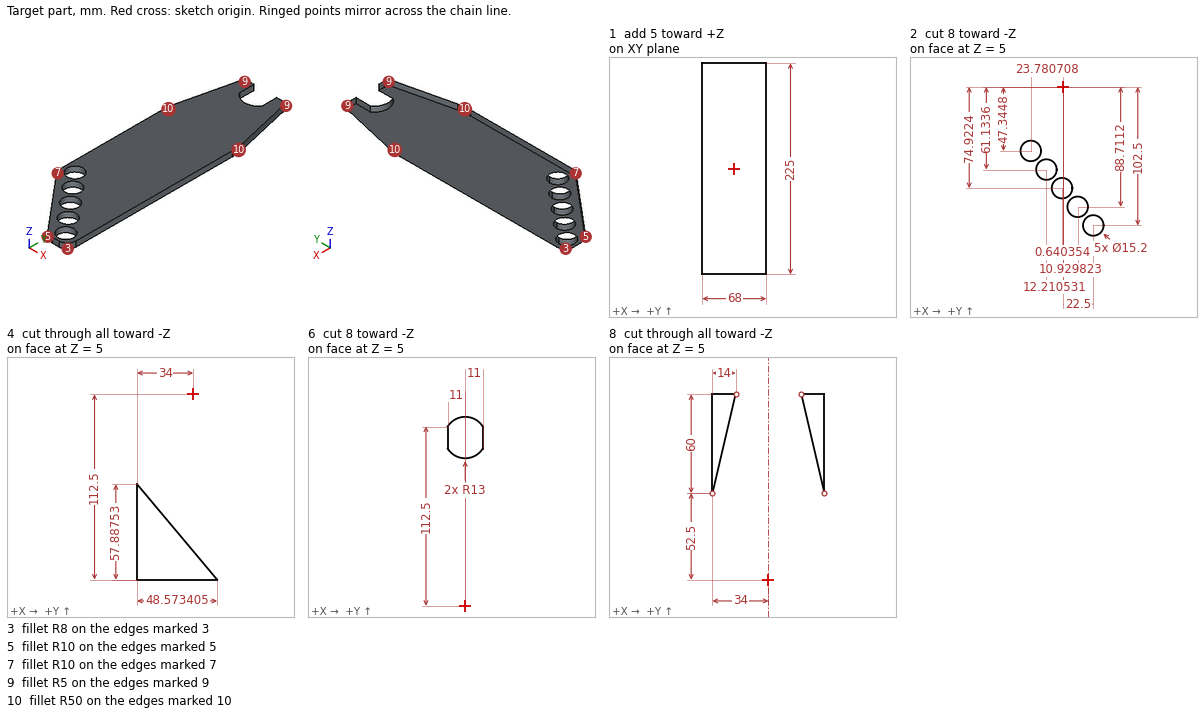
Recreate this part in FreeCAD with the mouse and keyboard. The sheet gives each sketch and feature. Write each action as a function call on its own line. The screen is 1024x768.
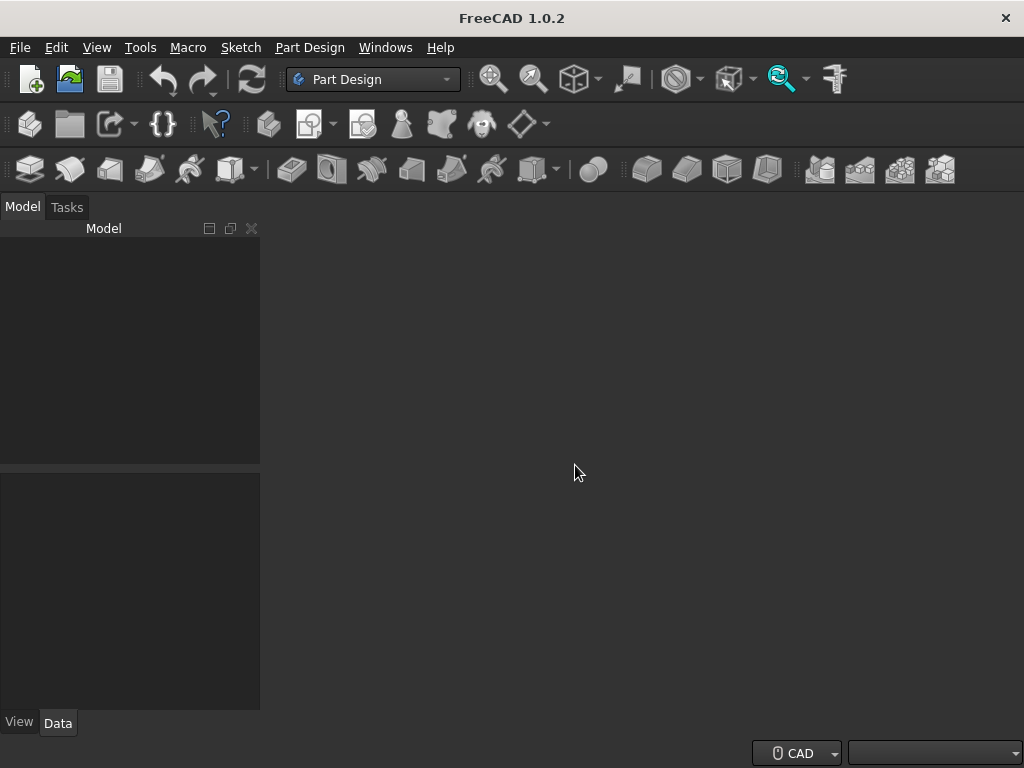
key(ctrl+n)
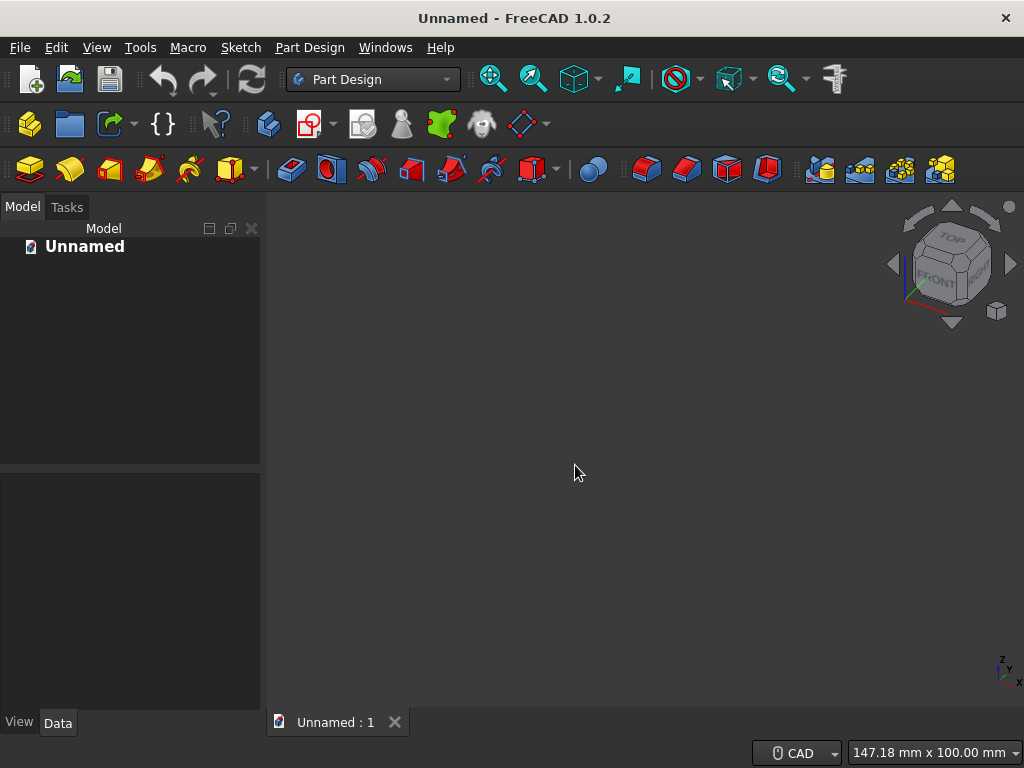
click(310, 124)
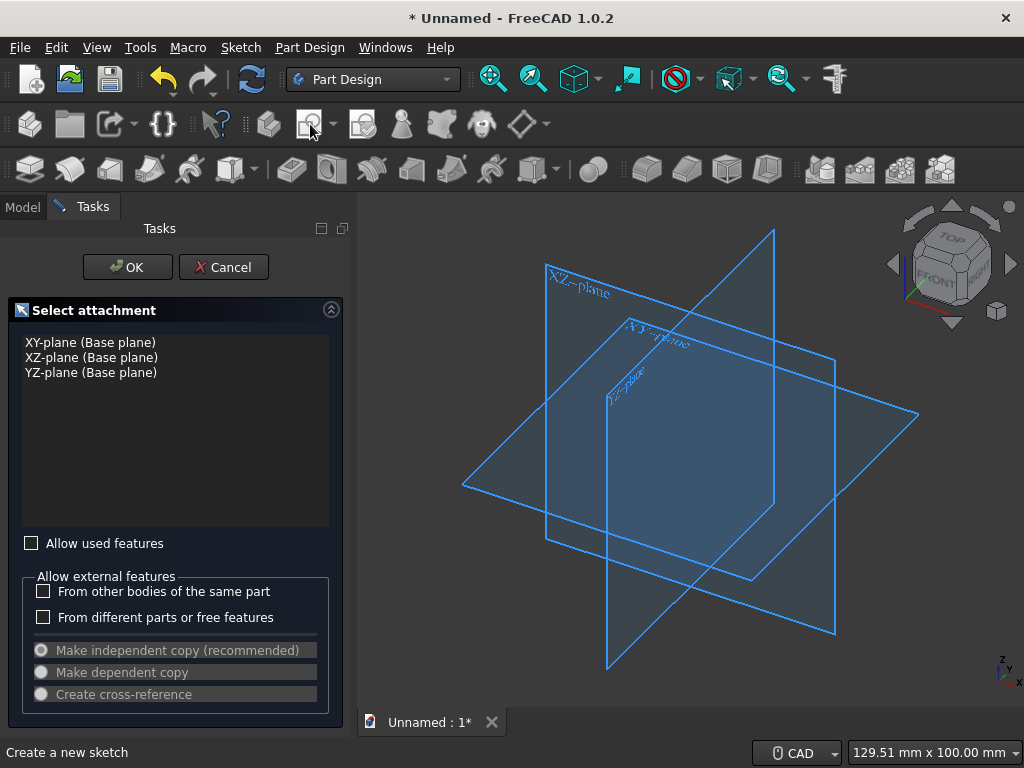
click(82, 342)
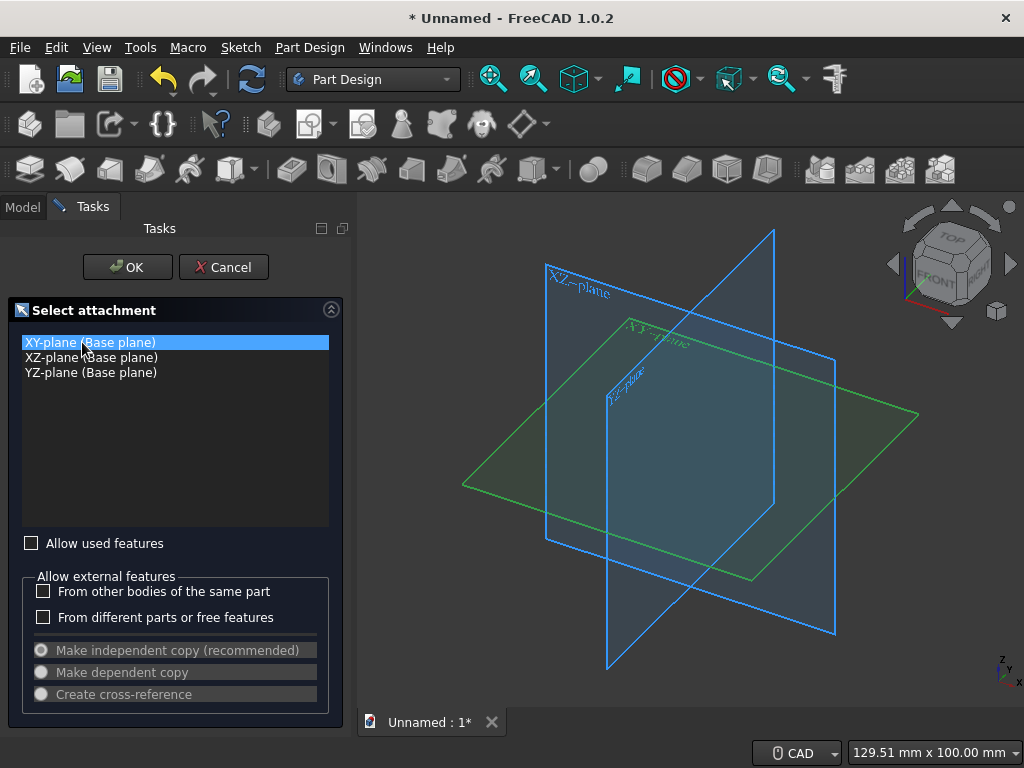
click(128, 267)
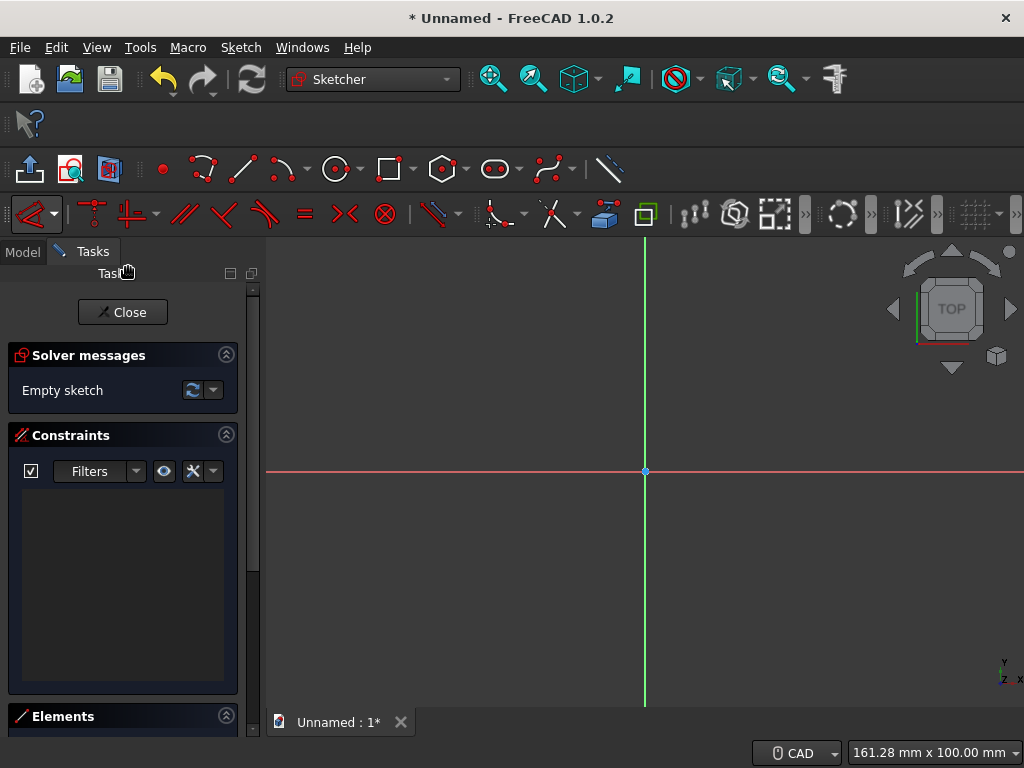
scroll(547, 472, down, 6)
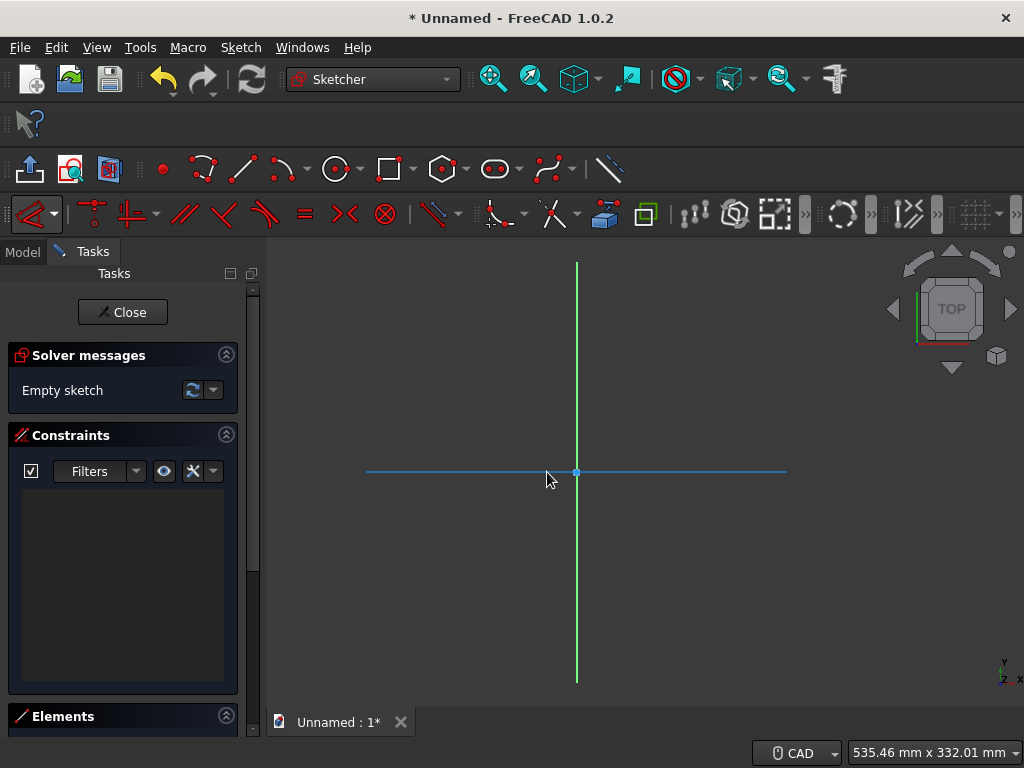
key(g)
key(v)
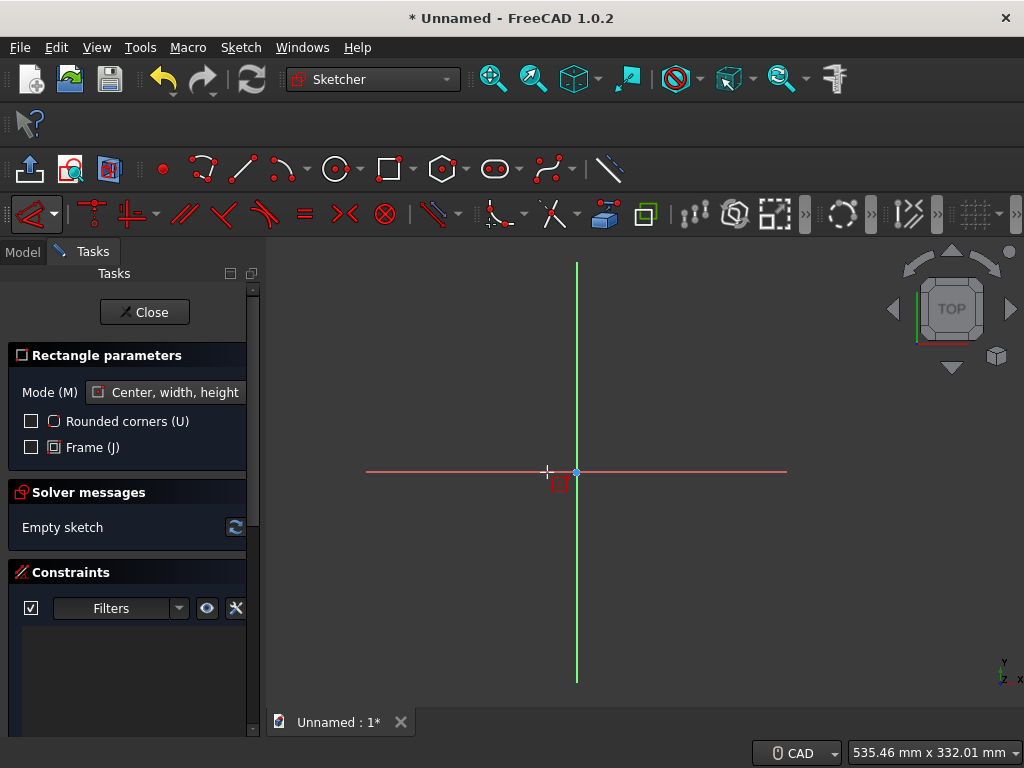
click(577, 472)
click(625, 313)
key(Escape)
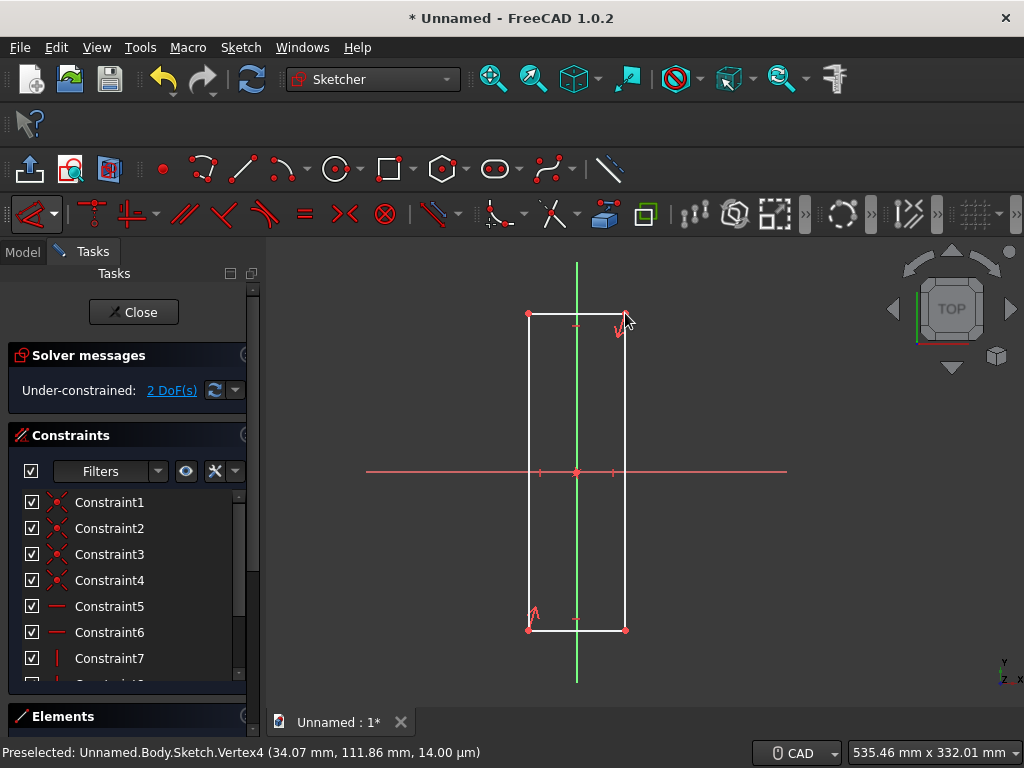
key(d)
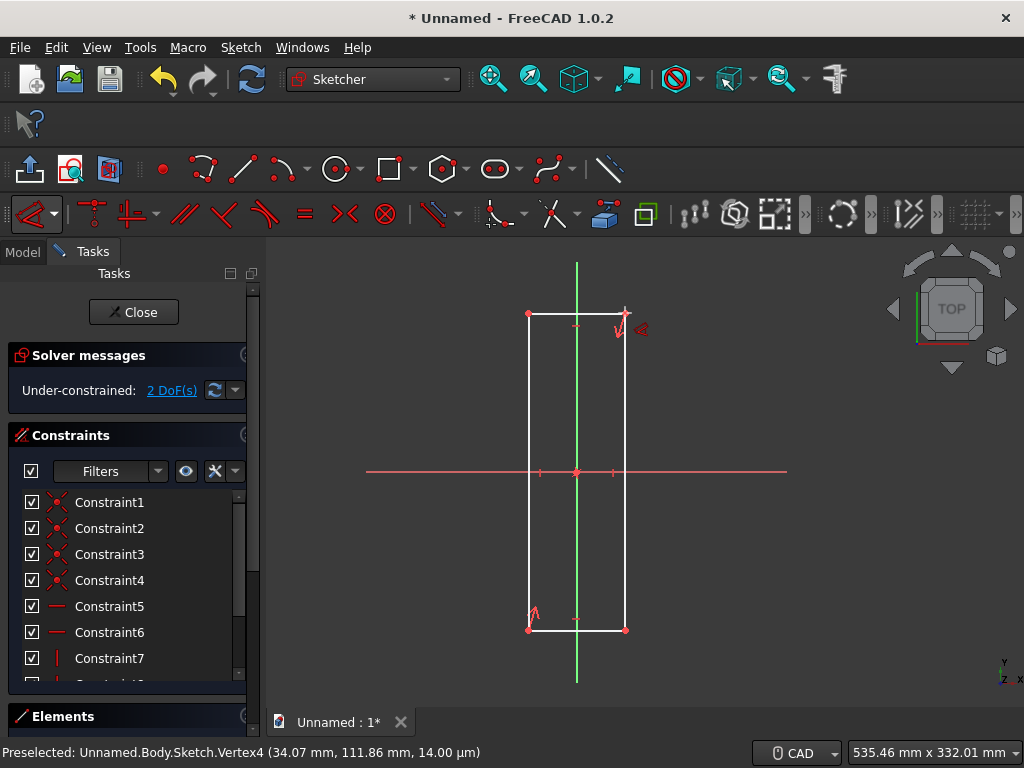
click(557, 631)
click(555, 665)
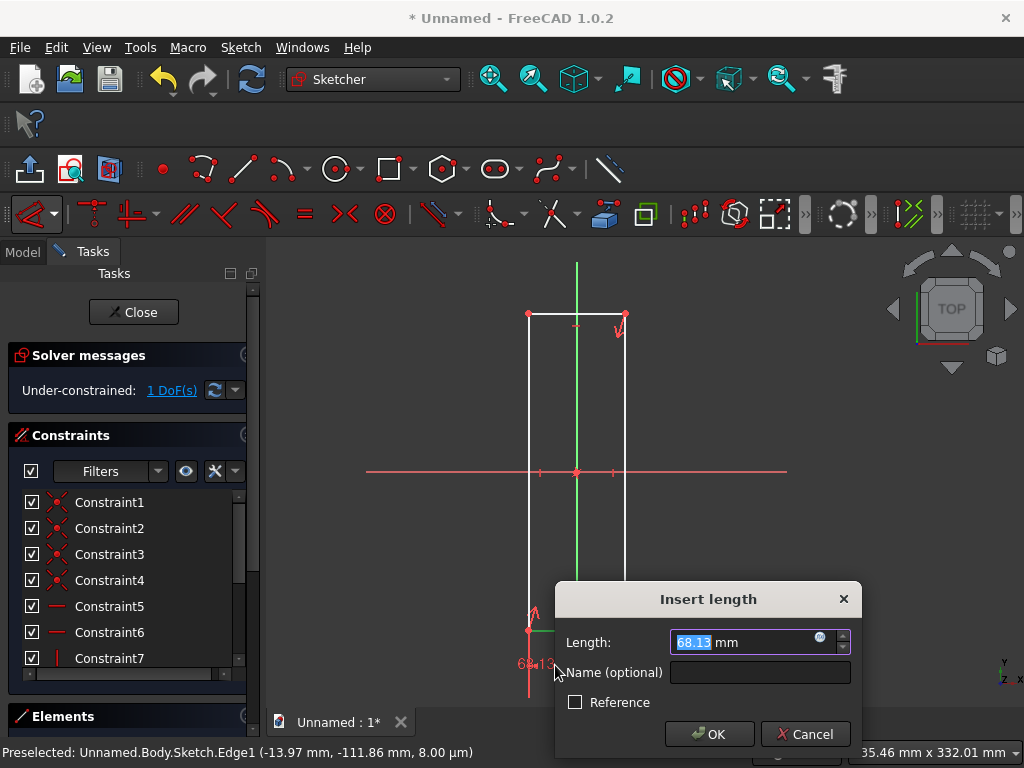
text(68)
key(Return)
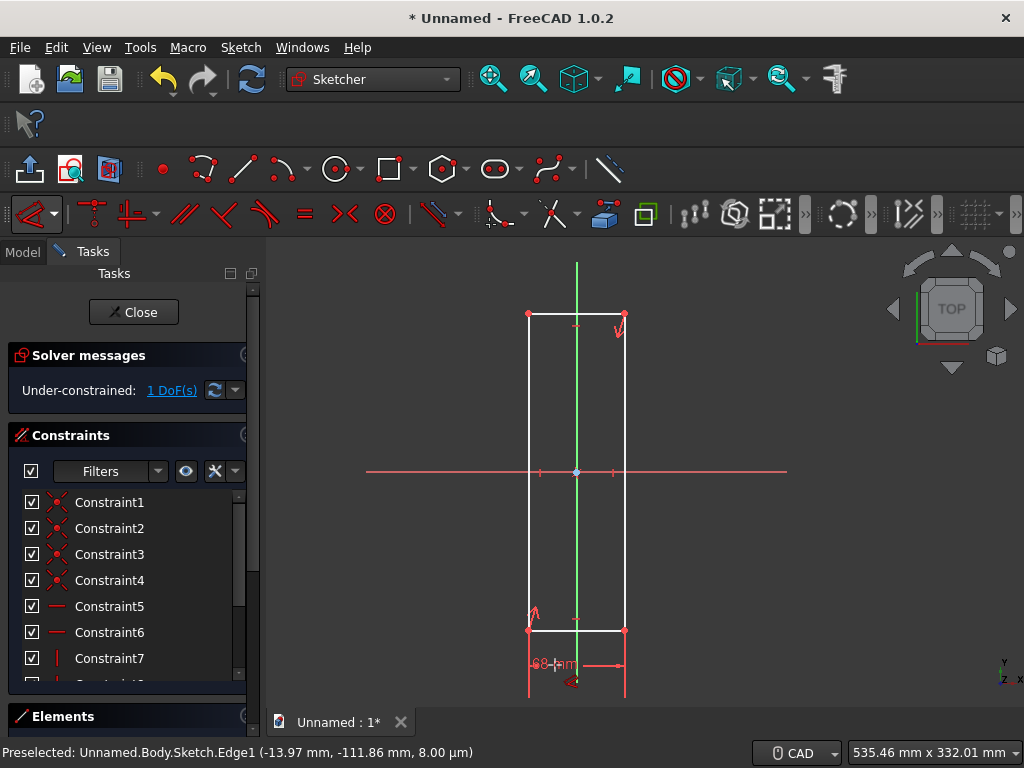
click(625, 536)
click(659, 400)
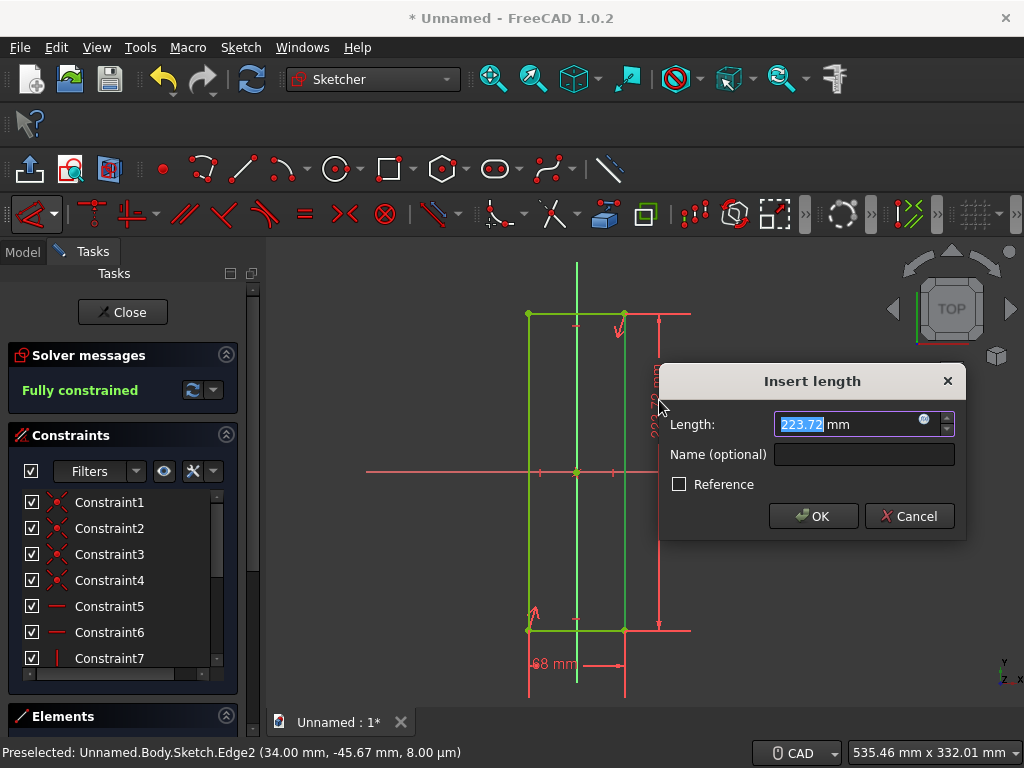
text(225)
key(Return)
key(Escape)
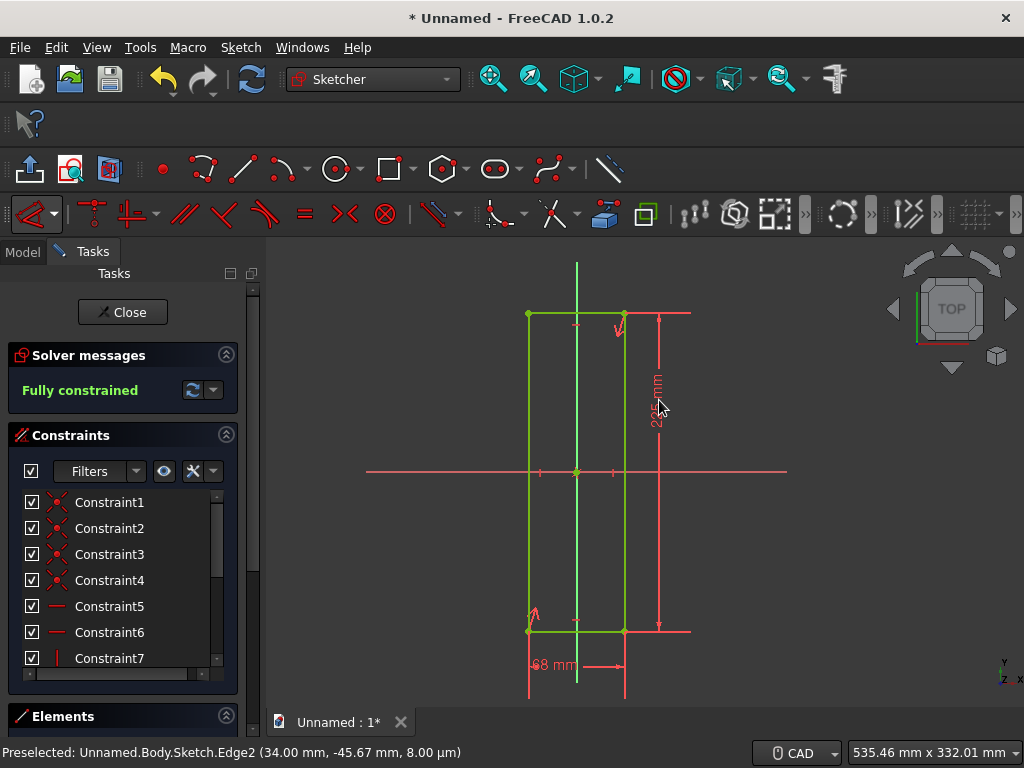
click(123, 312)